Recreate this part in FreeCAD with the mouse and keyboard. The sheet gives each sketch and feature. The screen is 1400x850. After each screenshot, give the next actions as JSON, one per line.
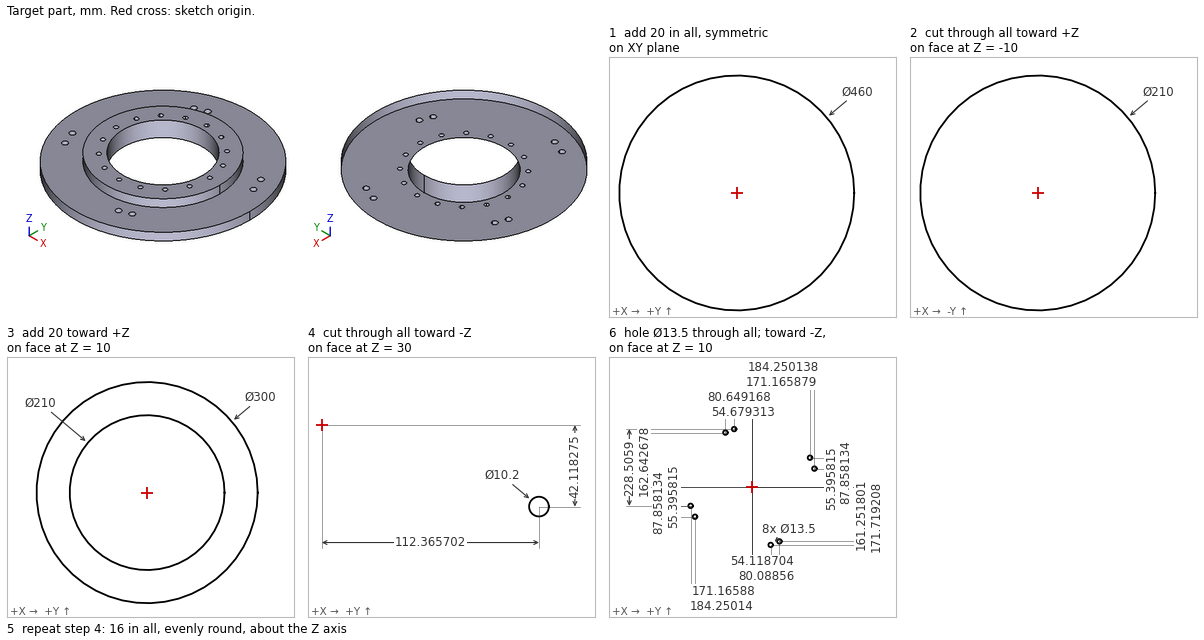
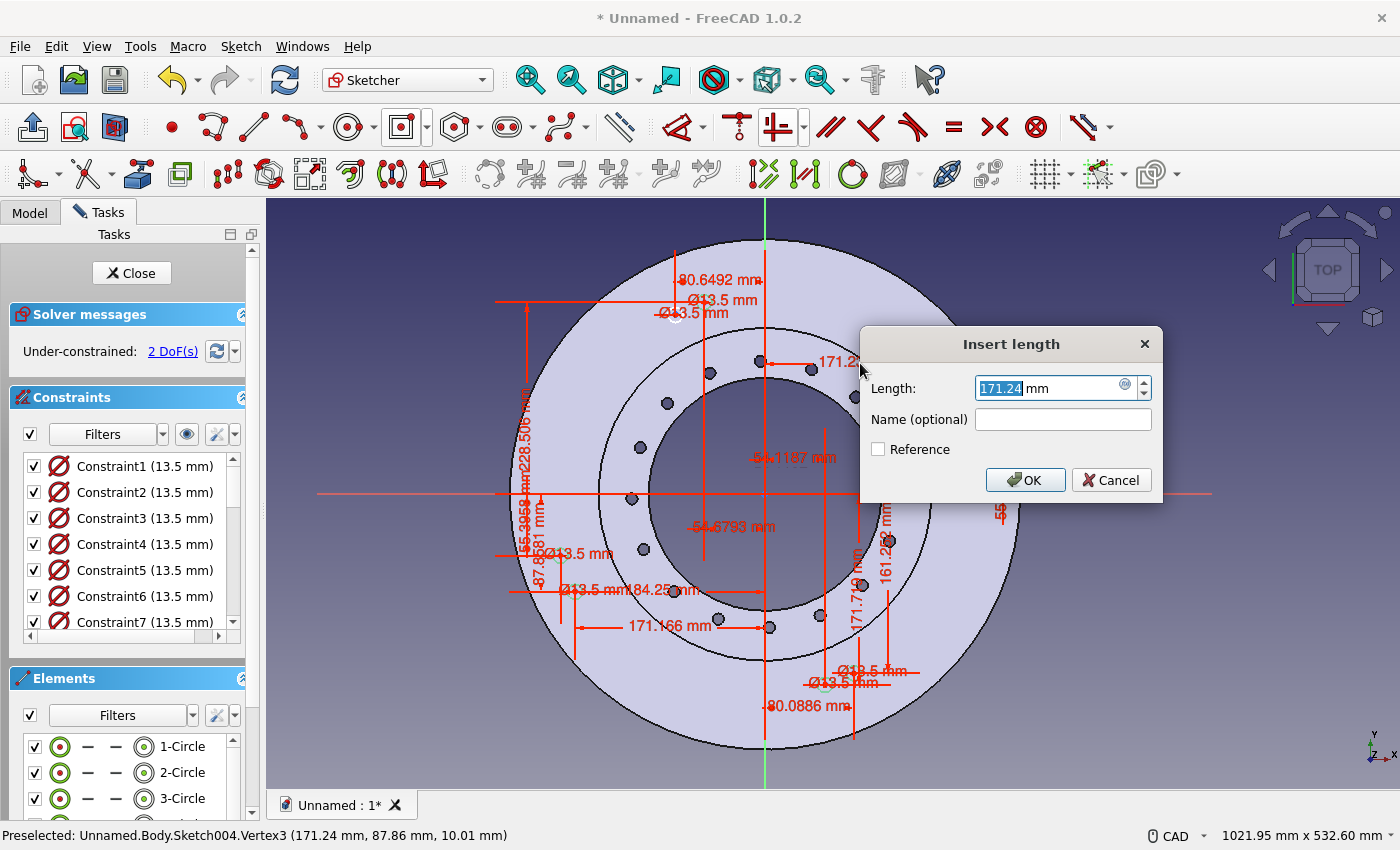
{"action": "type", "text": "171.165879"}
{"action": "key", "text": "Return"}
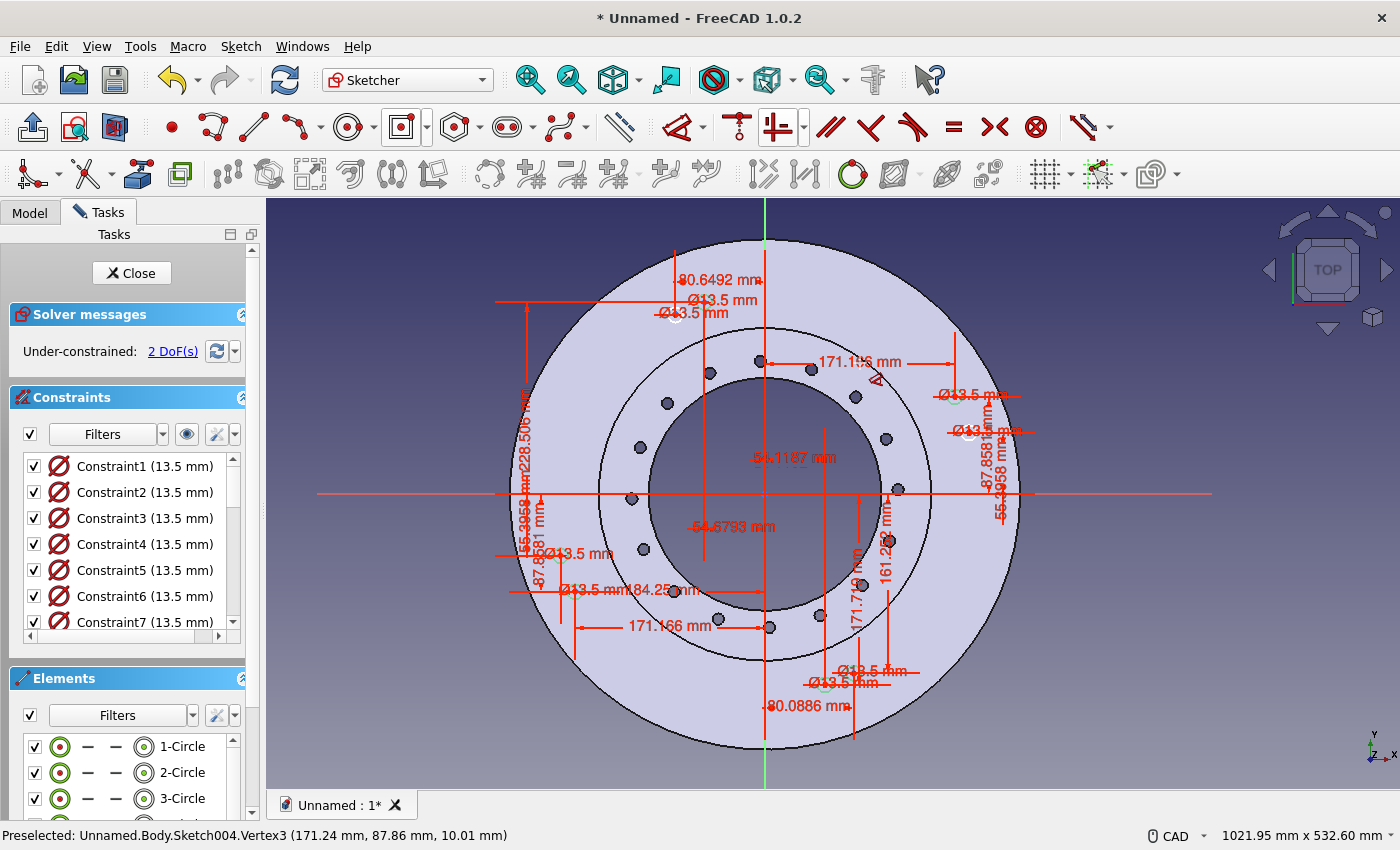
{"action": "left_click", "coordinate": [969, 433]}
{"action": "left_click", "coordinate": [867, 399]}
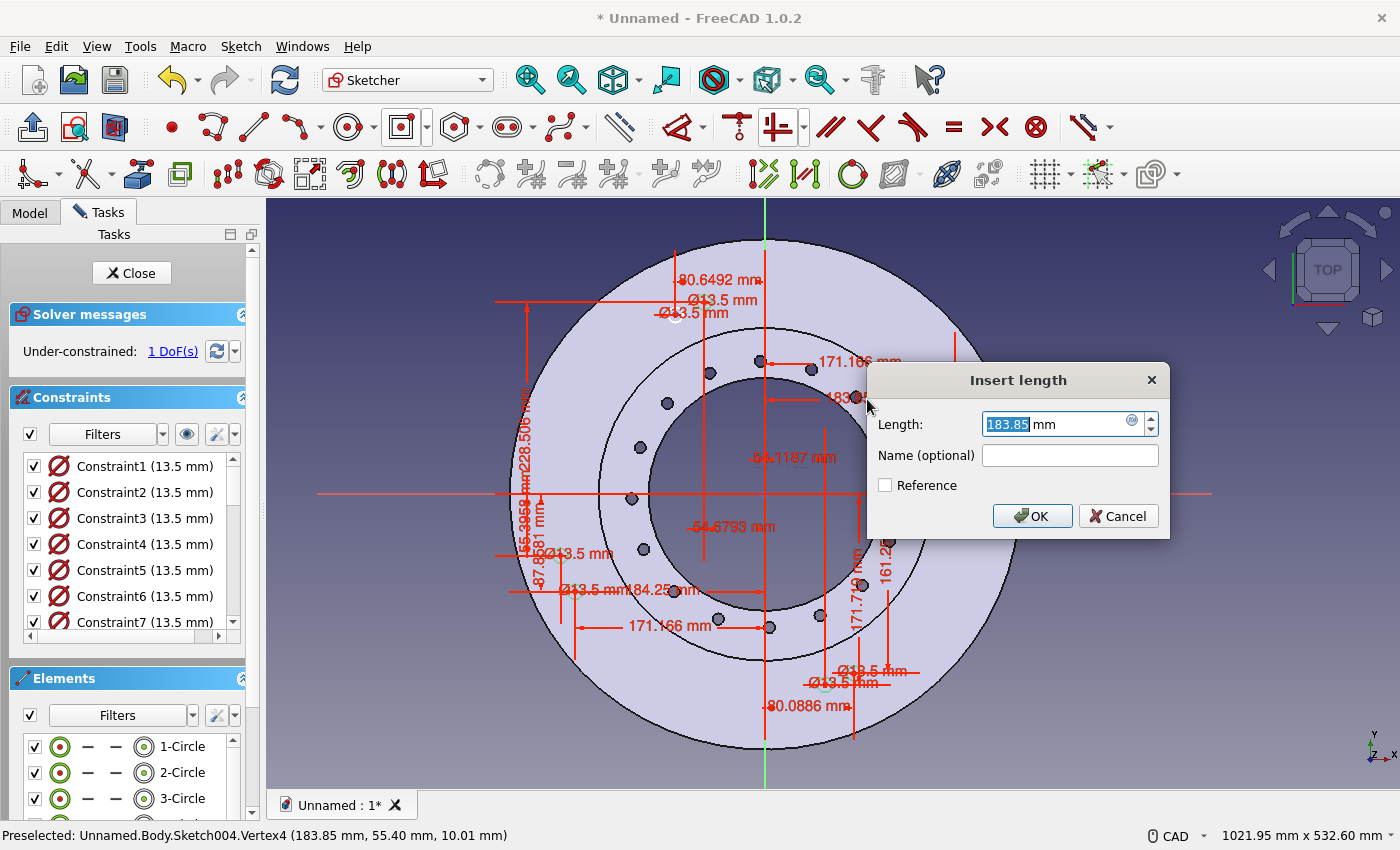
{"action": "type", "text": "184.250138"}
{"action": "key", "text": "Return"}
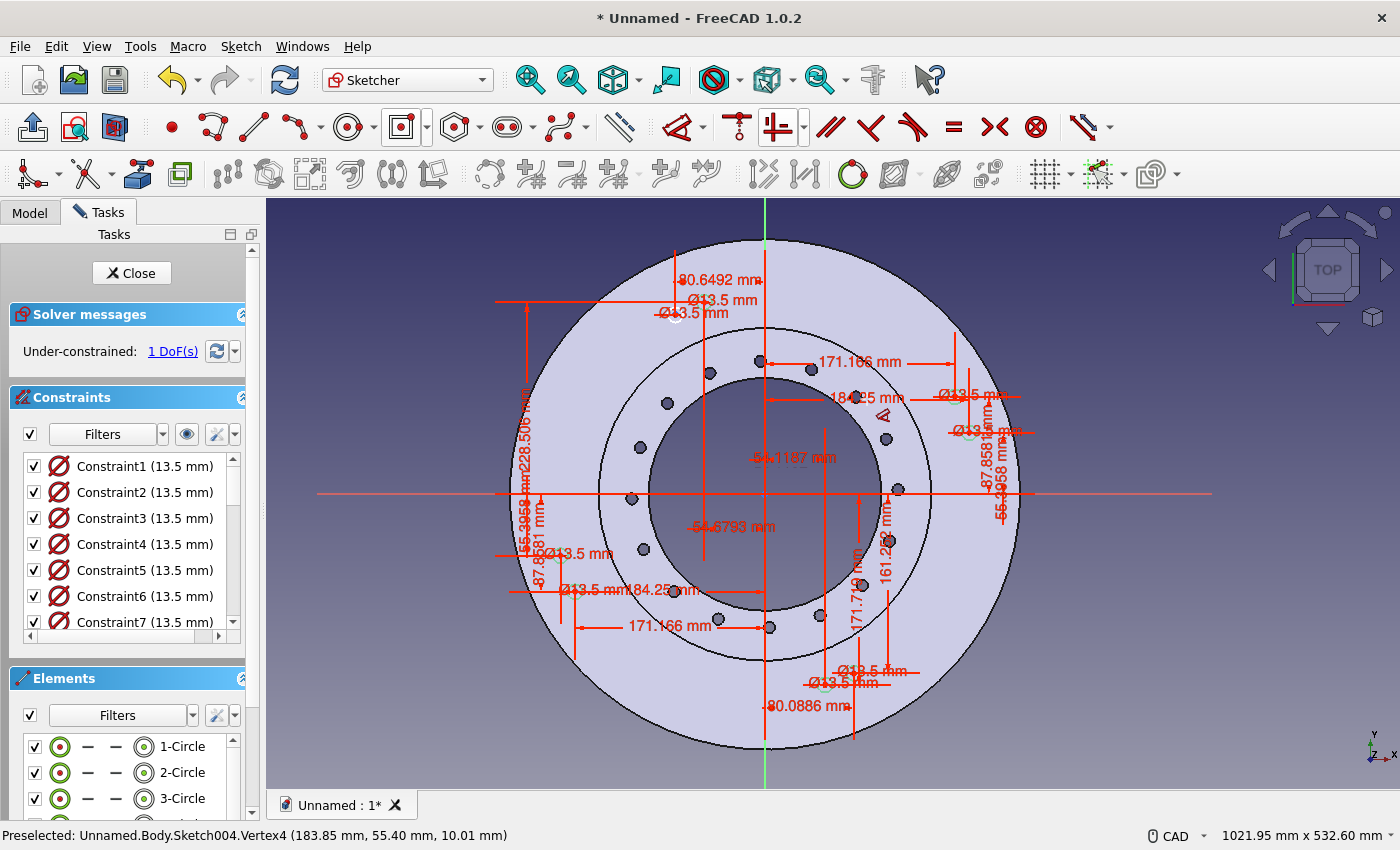
{"action": "left_click", "coordinate": [675, 315]}
{"action": "left_click", "coordinate": [641, 405]}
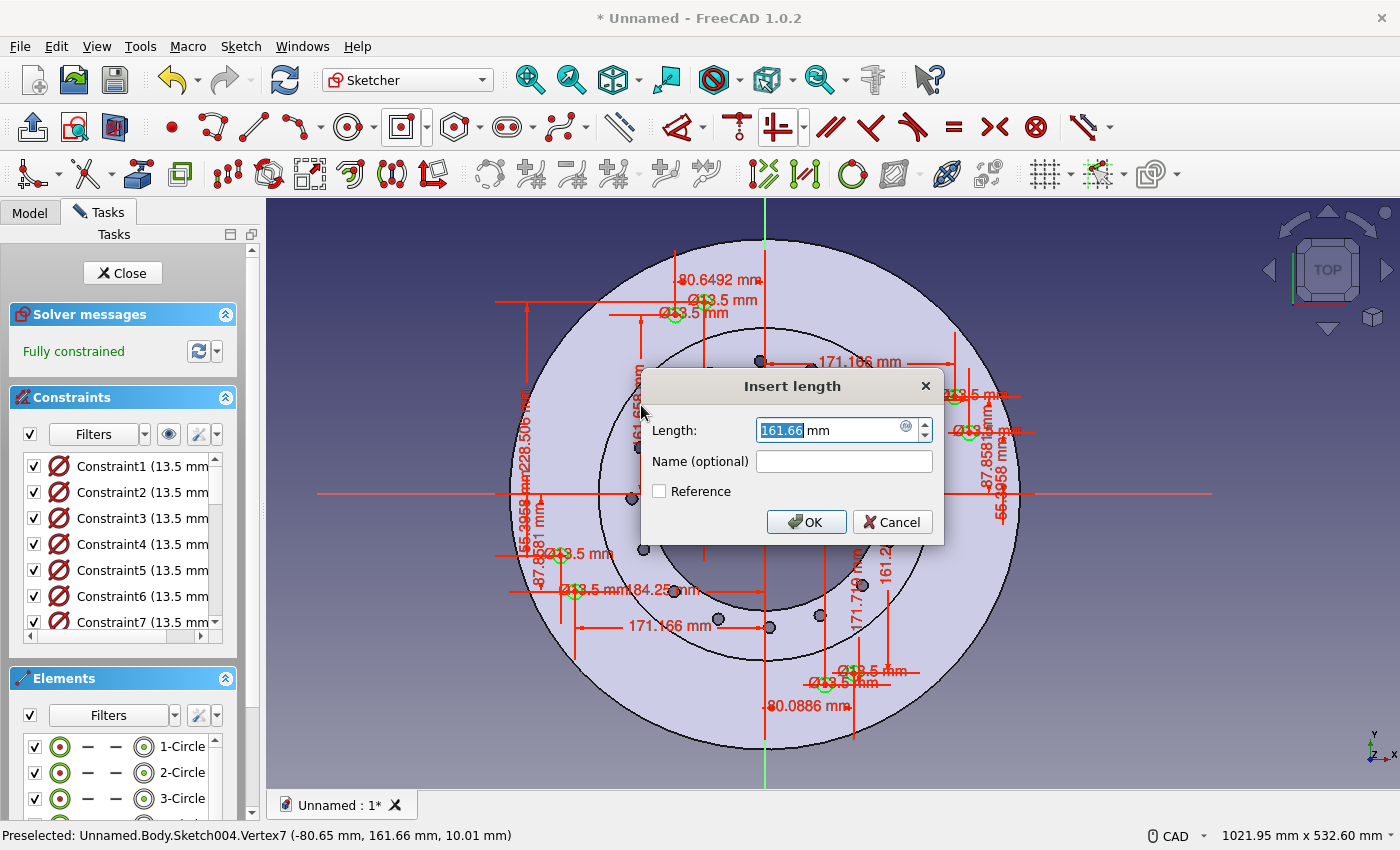
{"action": "type", "text": "162.642678"}
{"action": "key", "text": "Return"}
{"action": "key", "text": "Escape"}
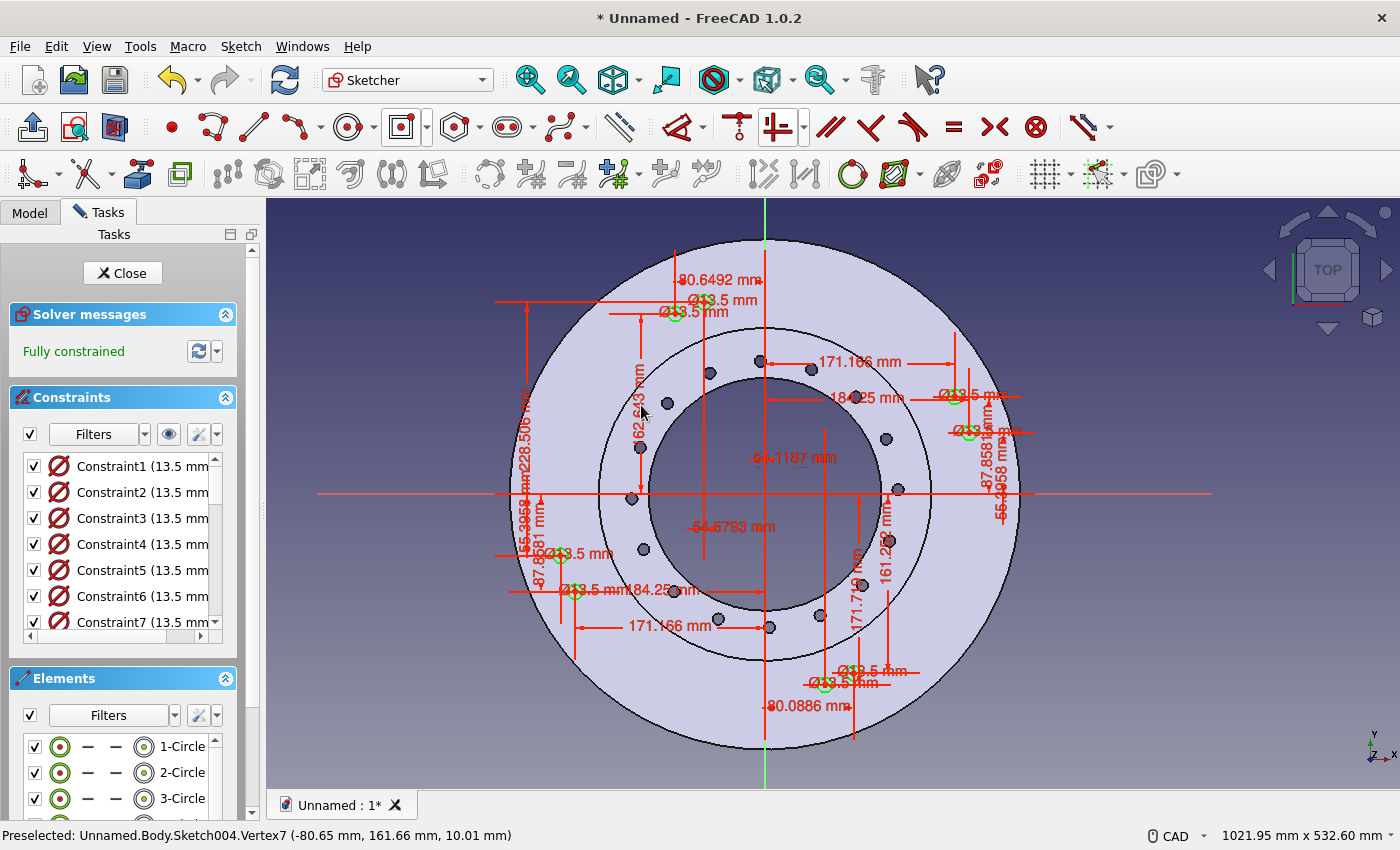
{"action": "left_click", "coordinate": [123, 273]}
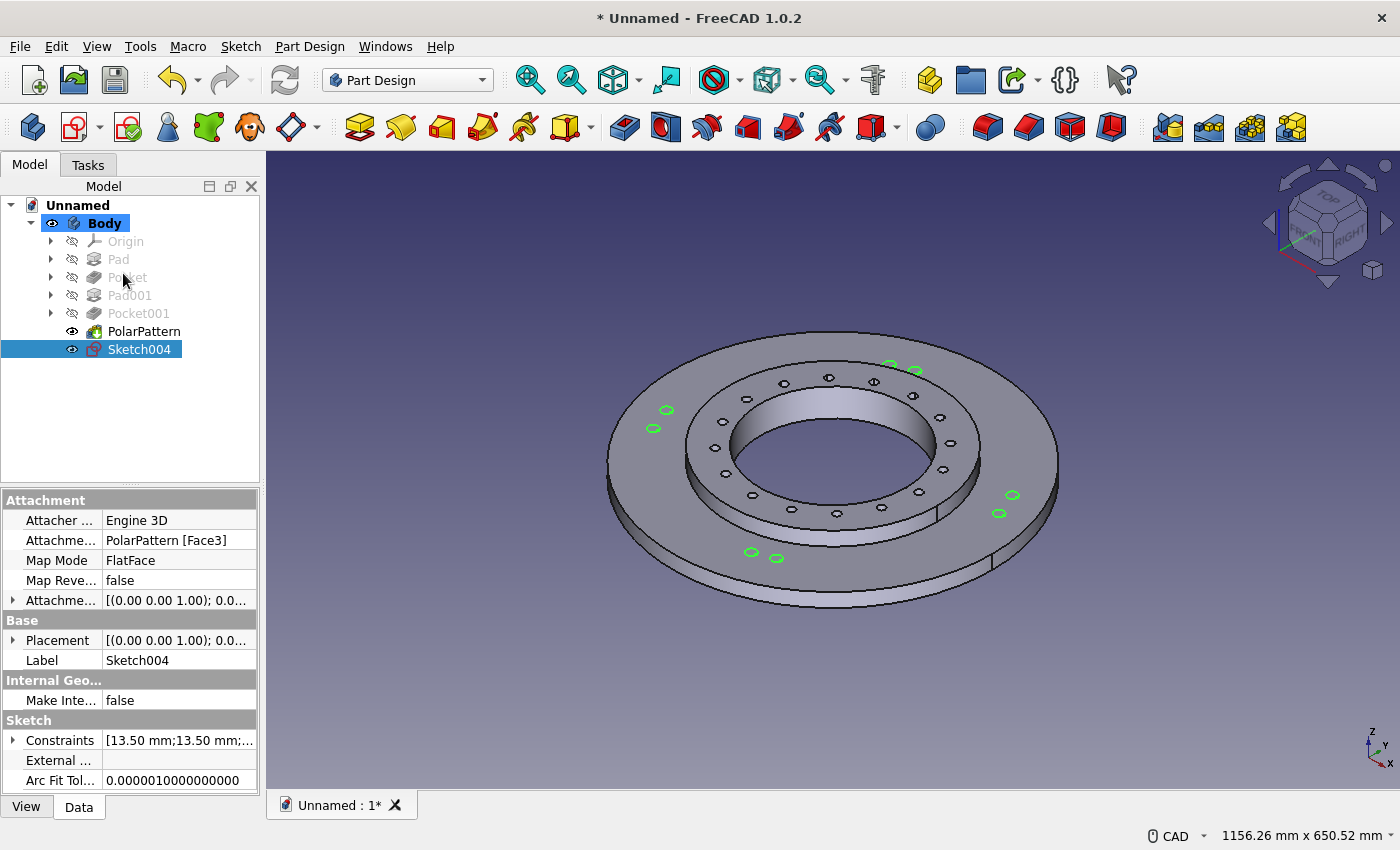
{"action": "left_click", "coordinate": [666, 128]}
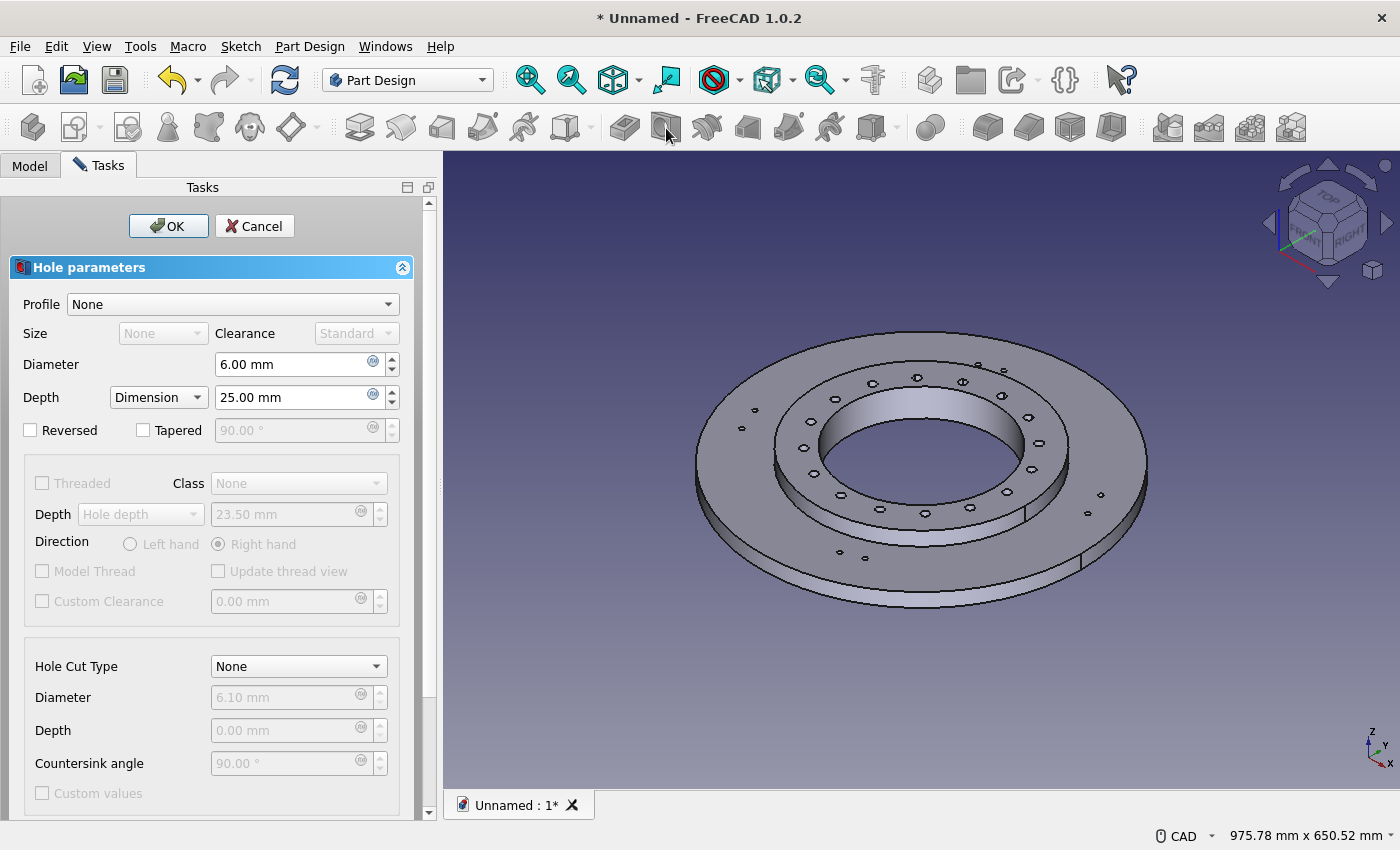
{"action": "triple_click", "coordinate": [300, 364]}